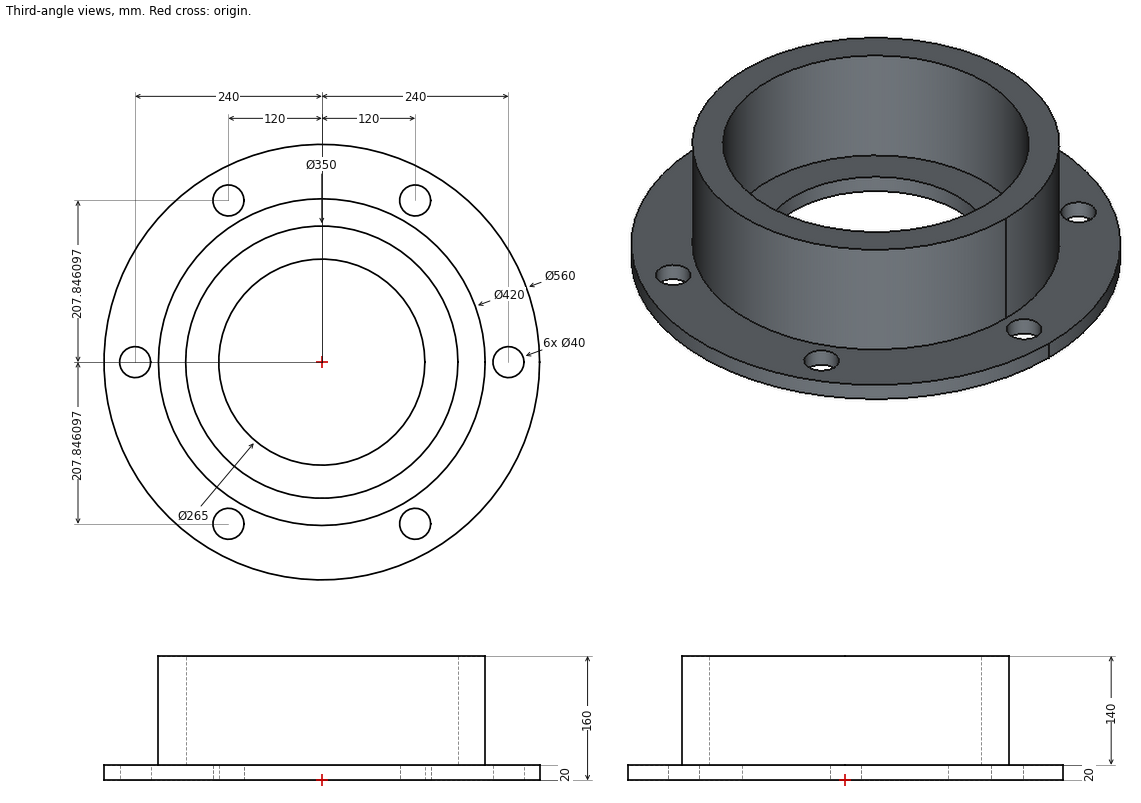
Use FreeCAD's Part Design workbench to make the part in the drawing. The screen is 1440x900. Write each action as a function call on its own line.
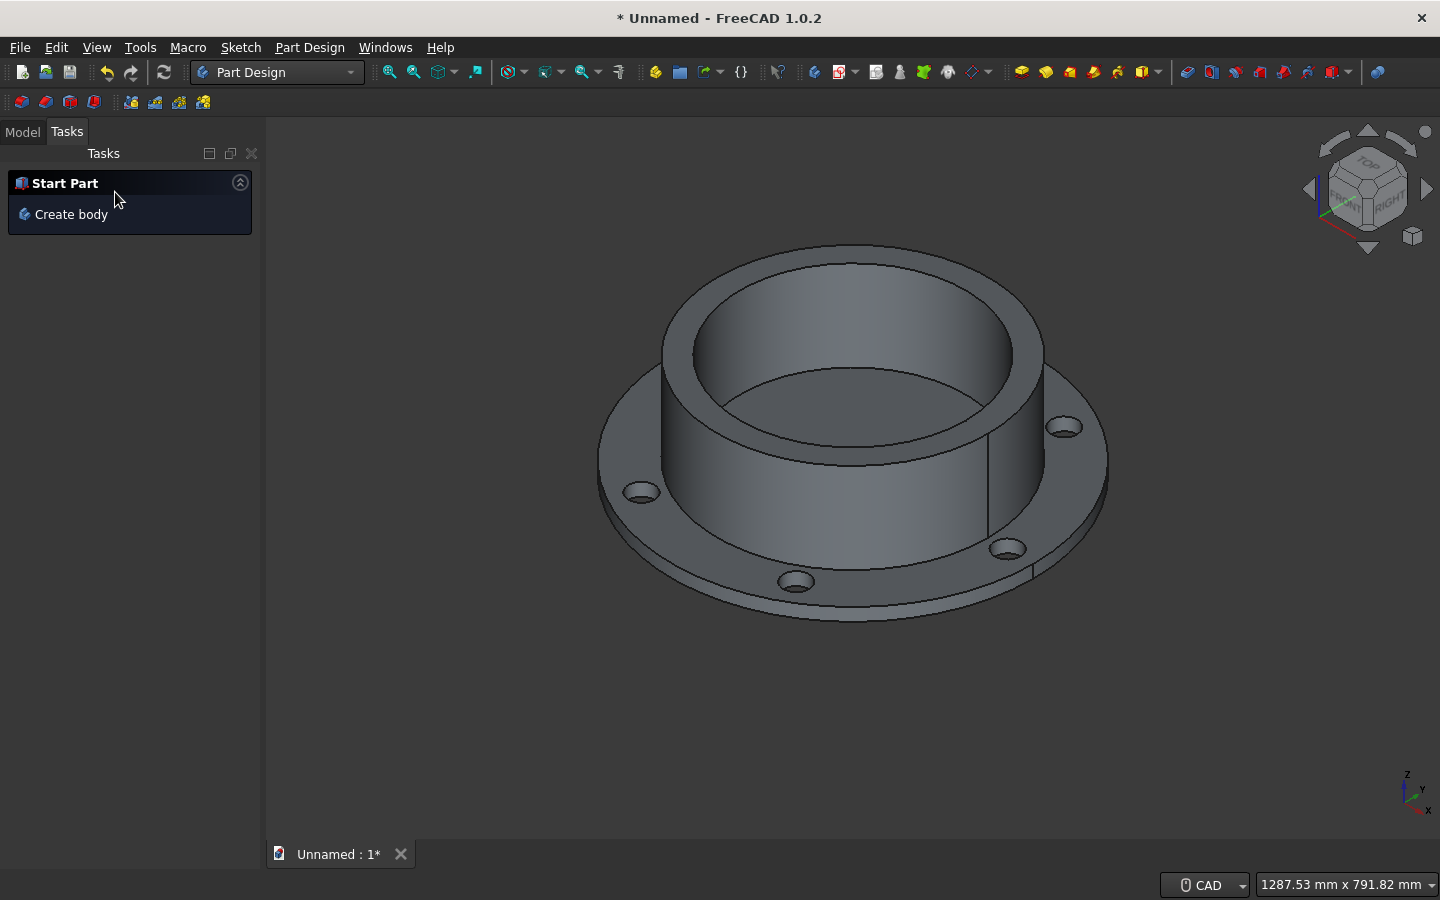
key(5)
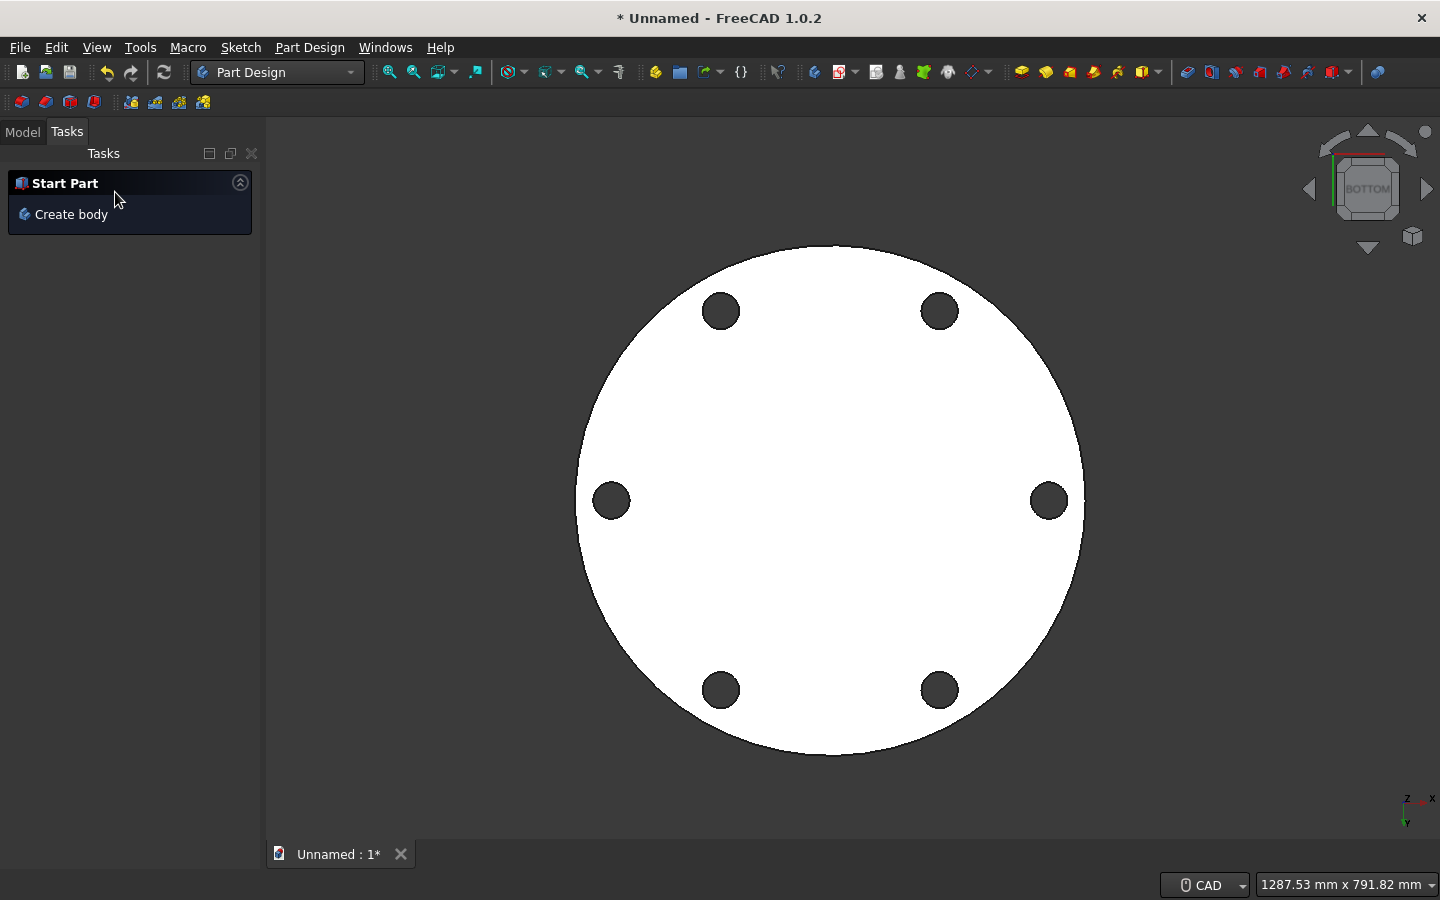
click(830, 500)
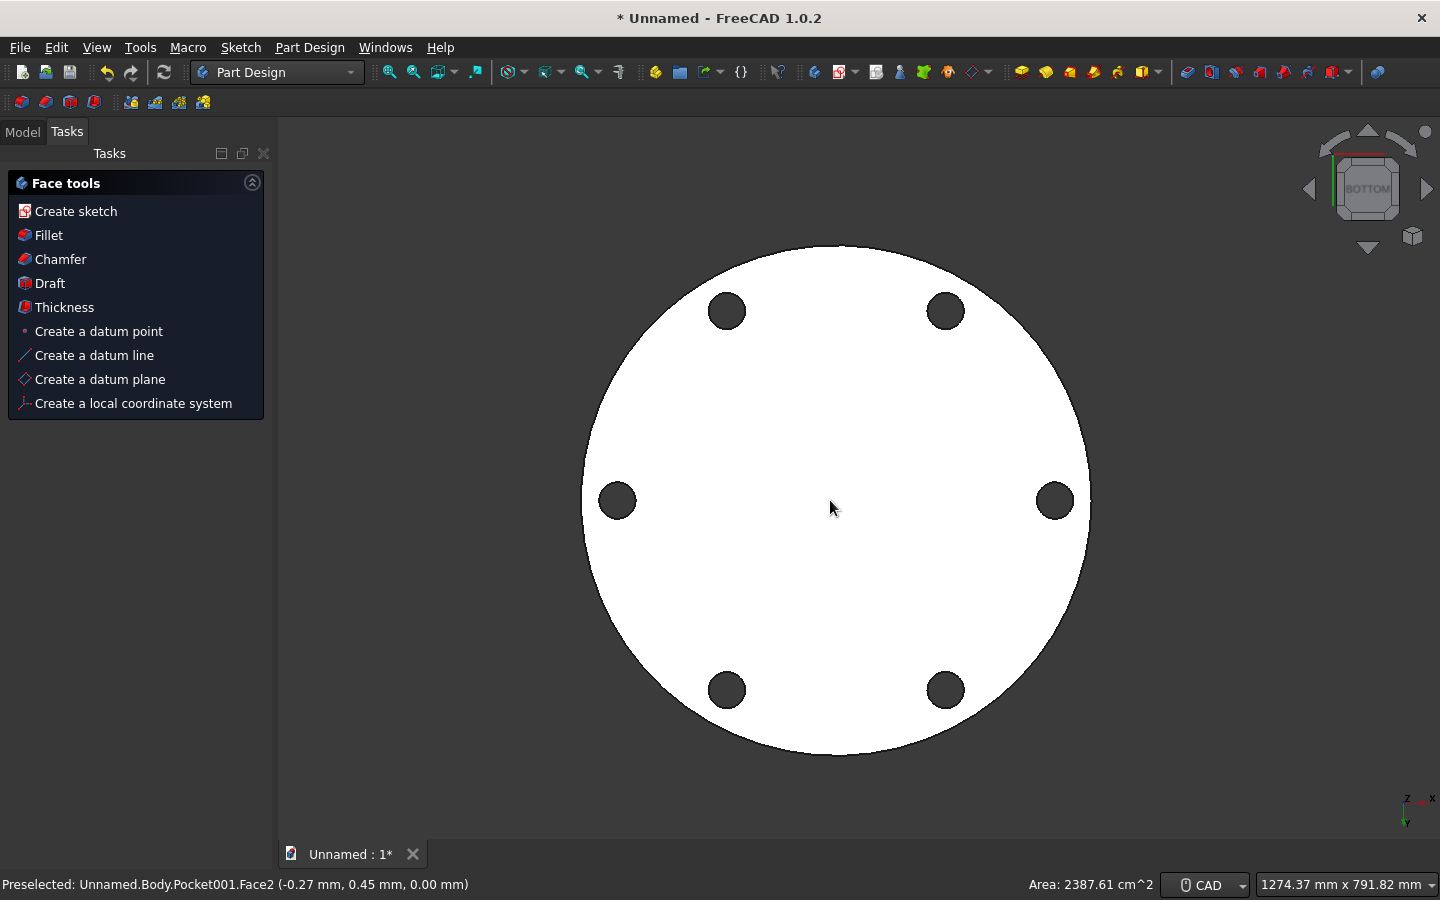
click(840, 72)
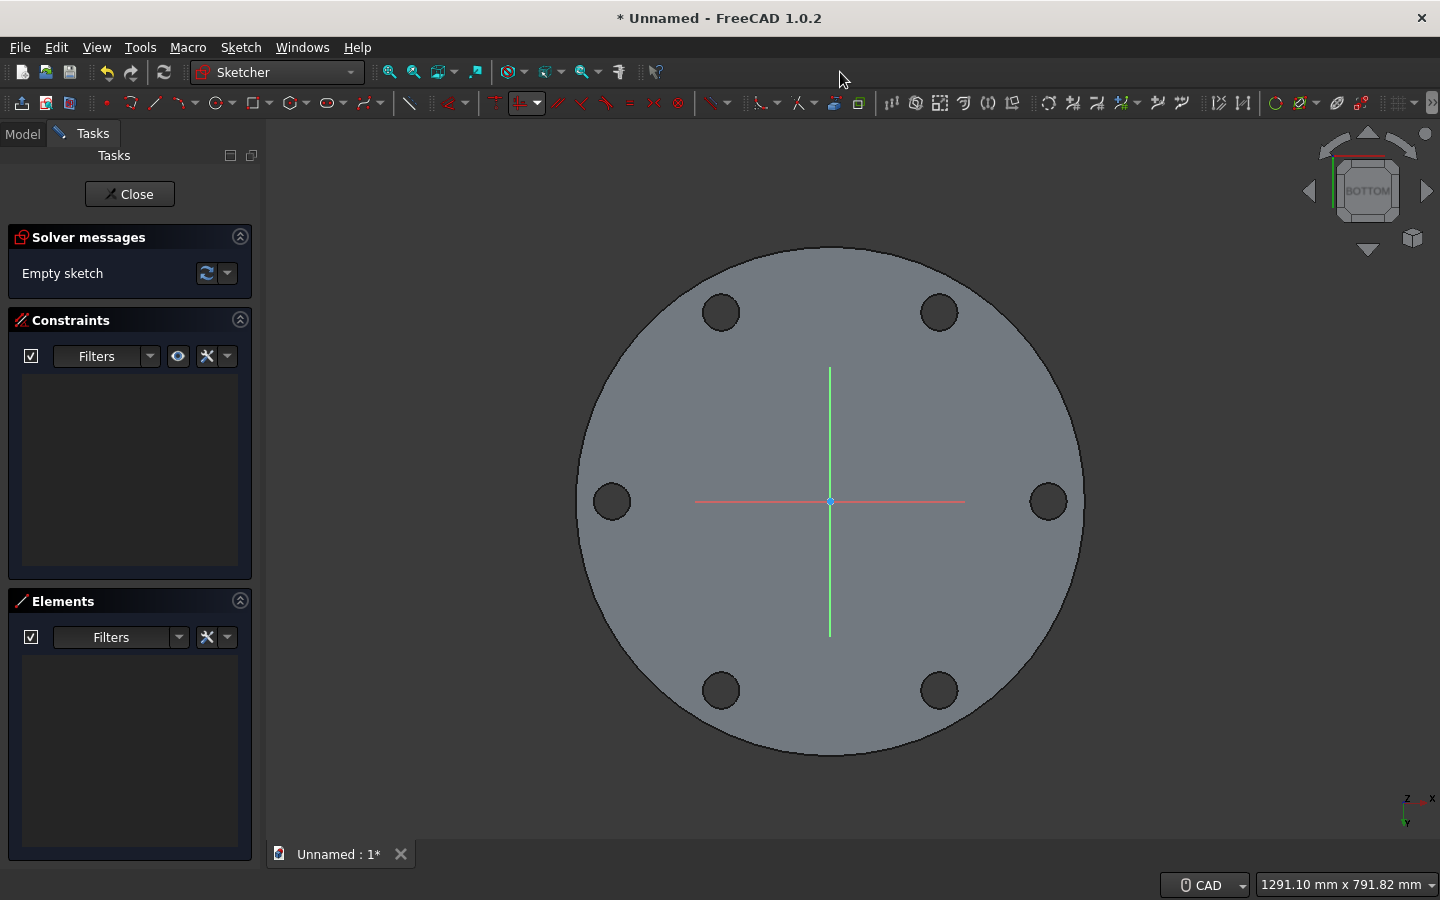
scroll(886, 529, up, 3)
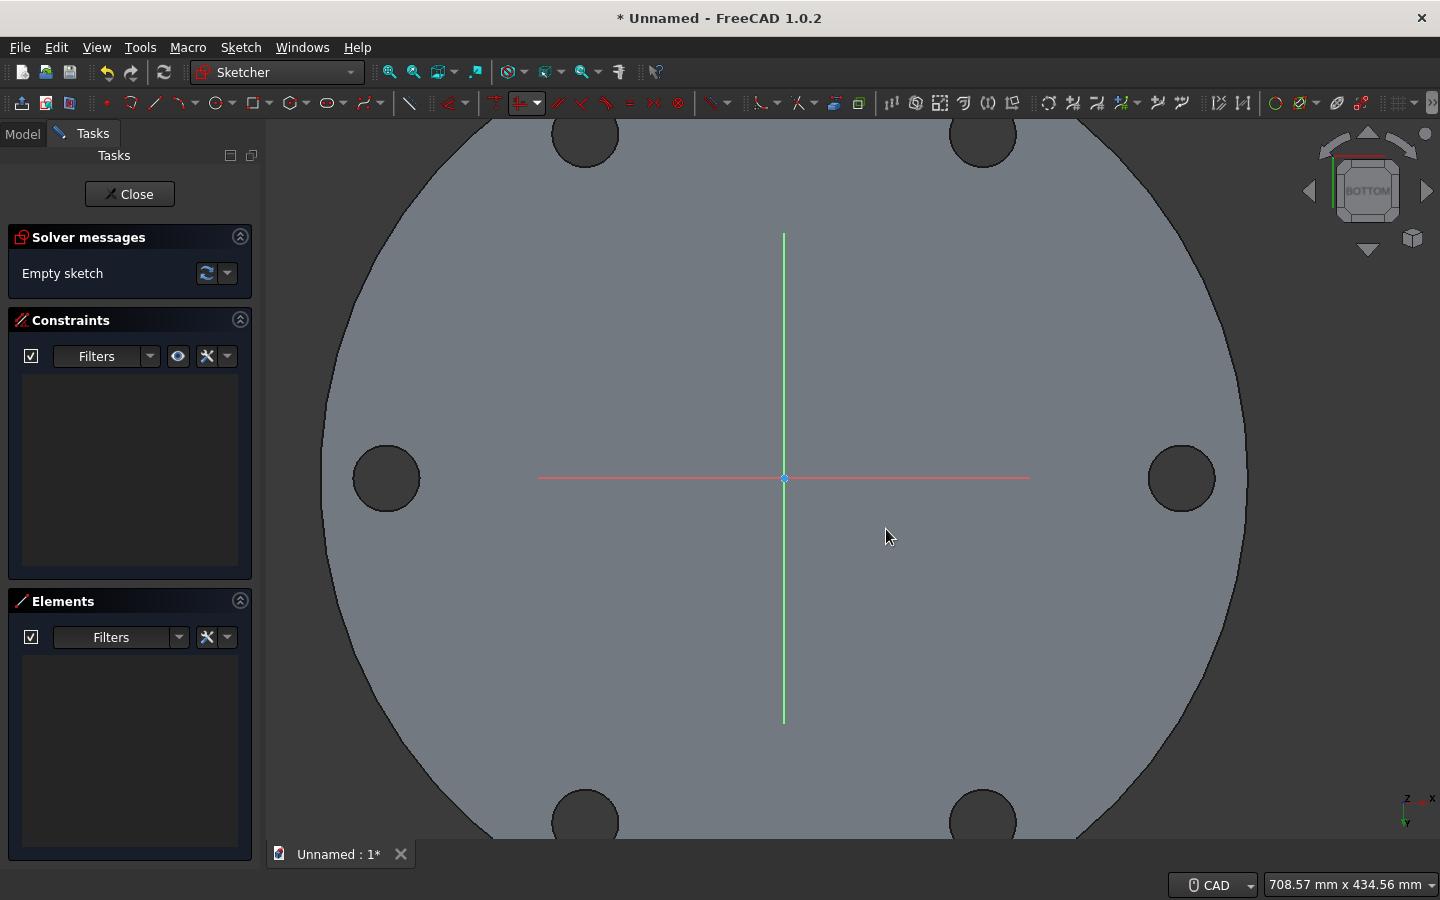
click(216, 104)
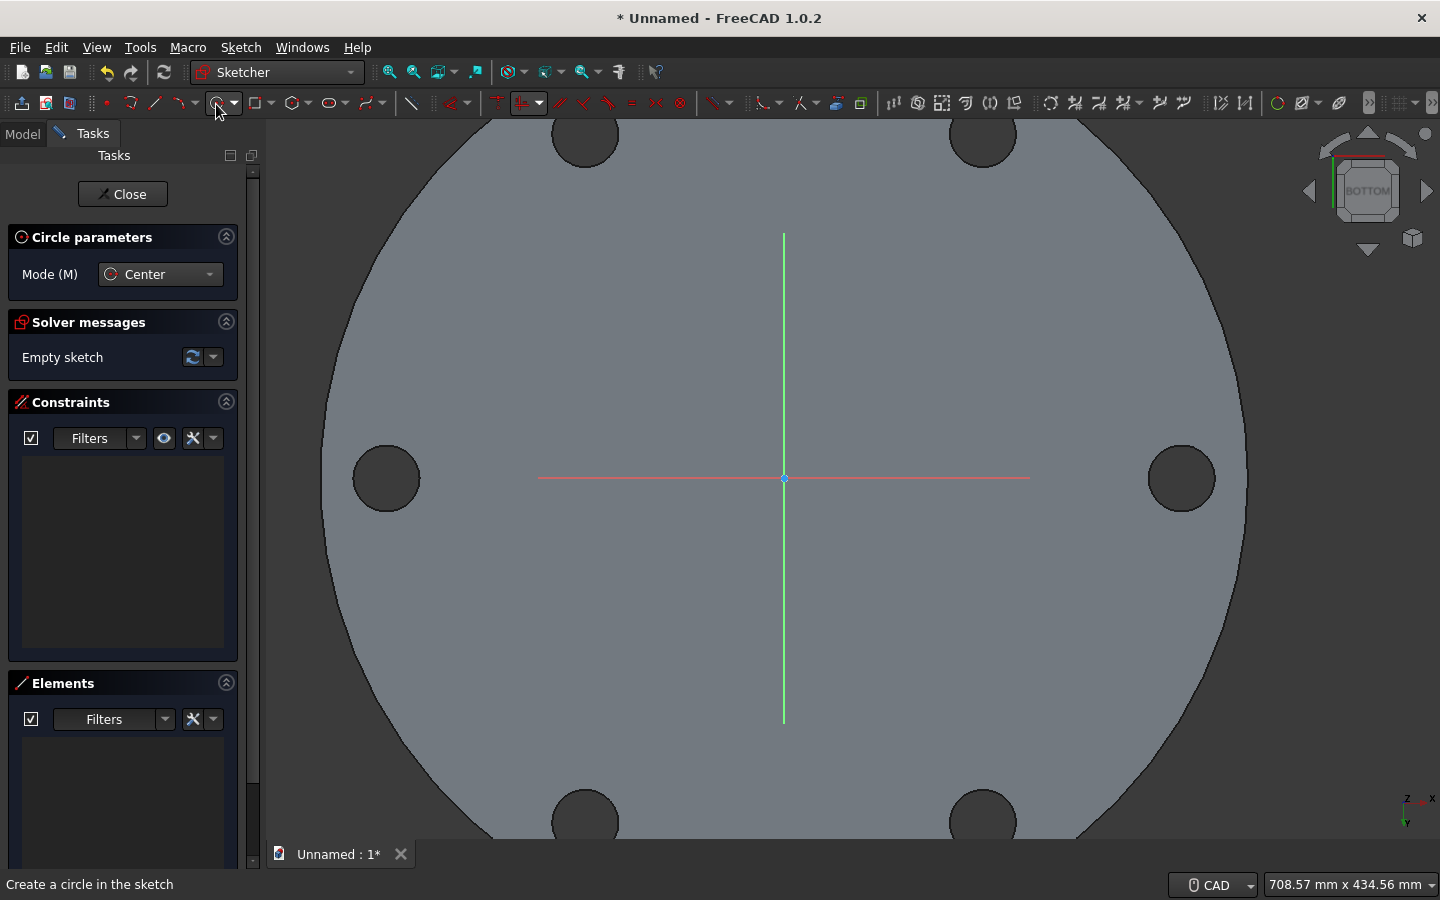
click(784, 478)
click(939, 323)
key(Escape)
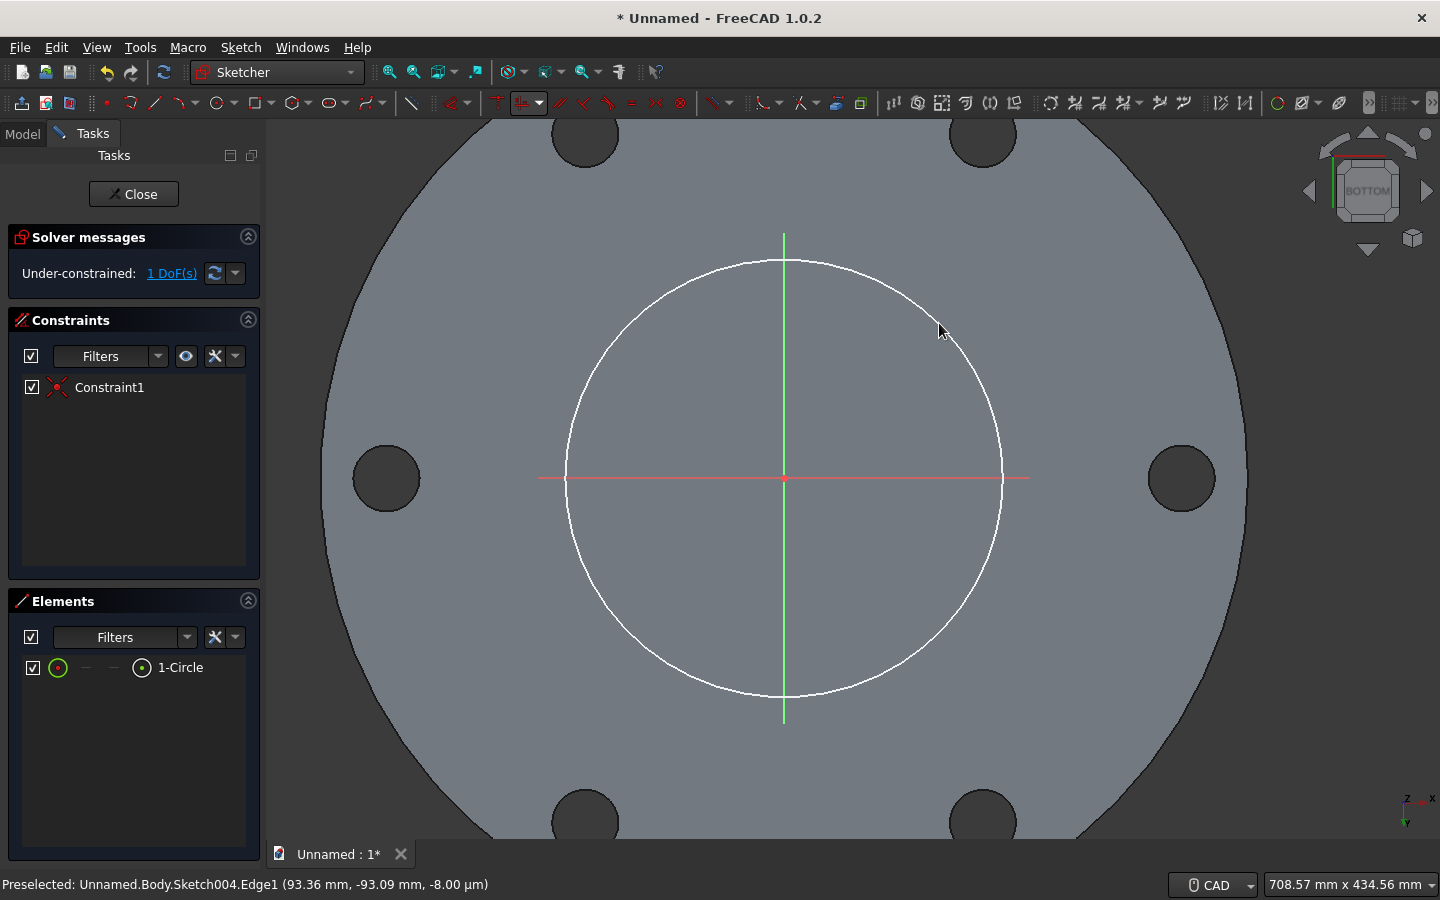
key(d)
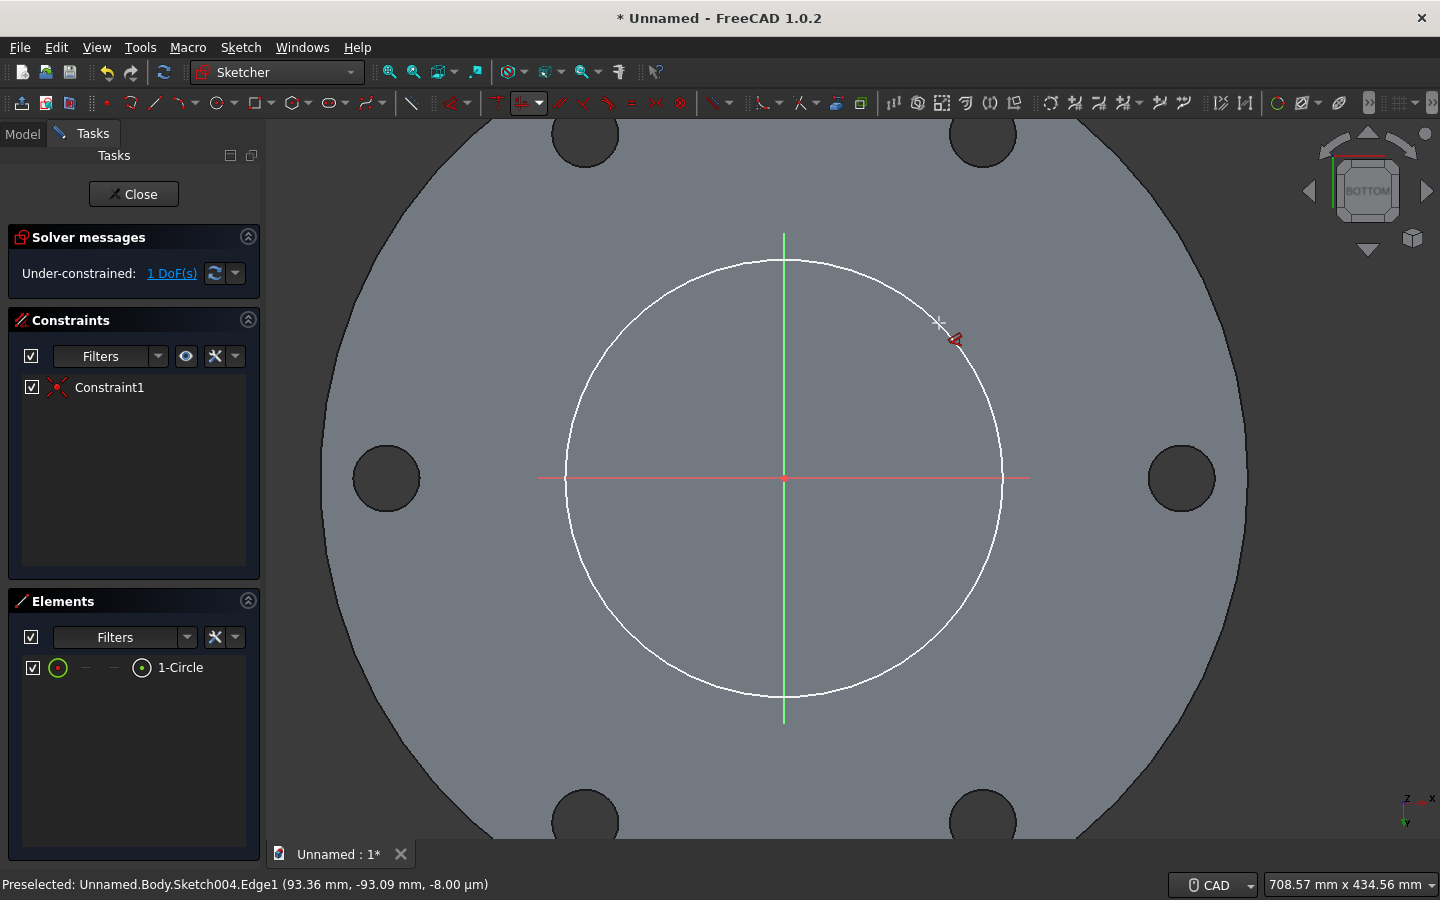
click(938, 323)
click(961, 300)